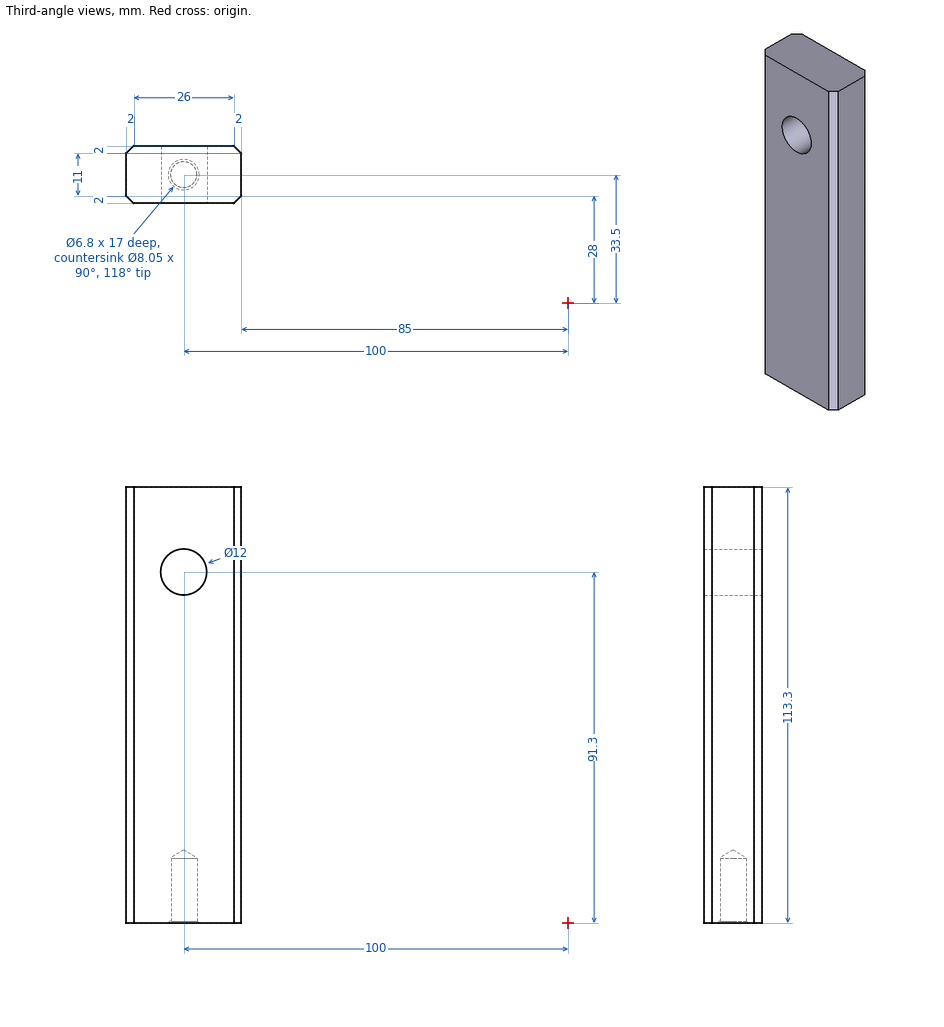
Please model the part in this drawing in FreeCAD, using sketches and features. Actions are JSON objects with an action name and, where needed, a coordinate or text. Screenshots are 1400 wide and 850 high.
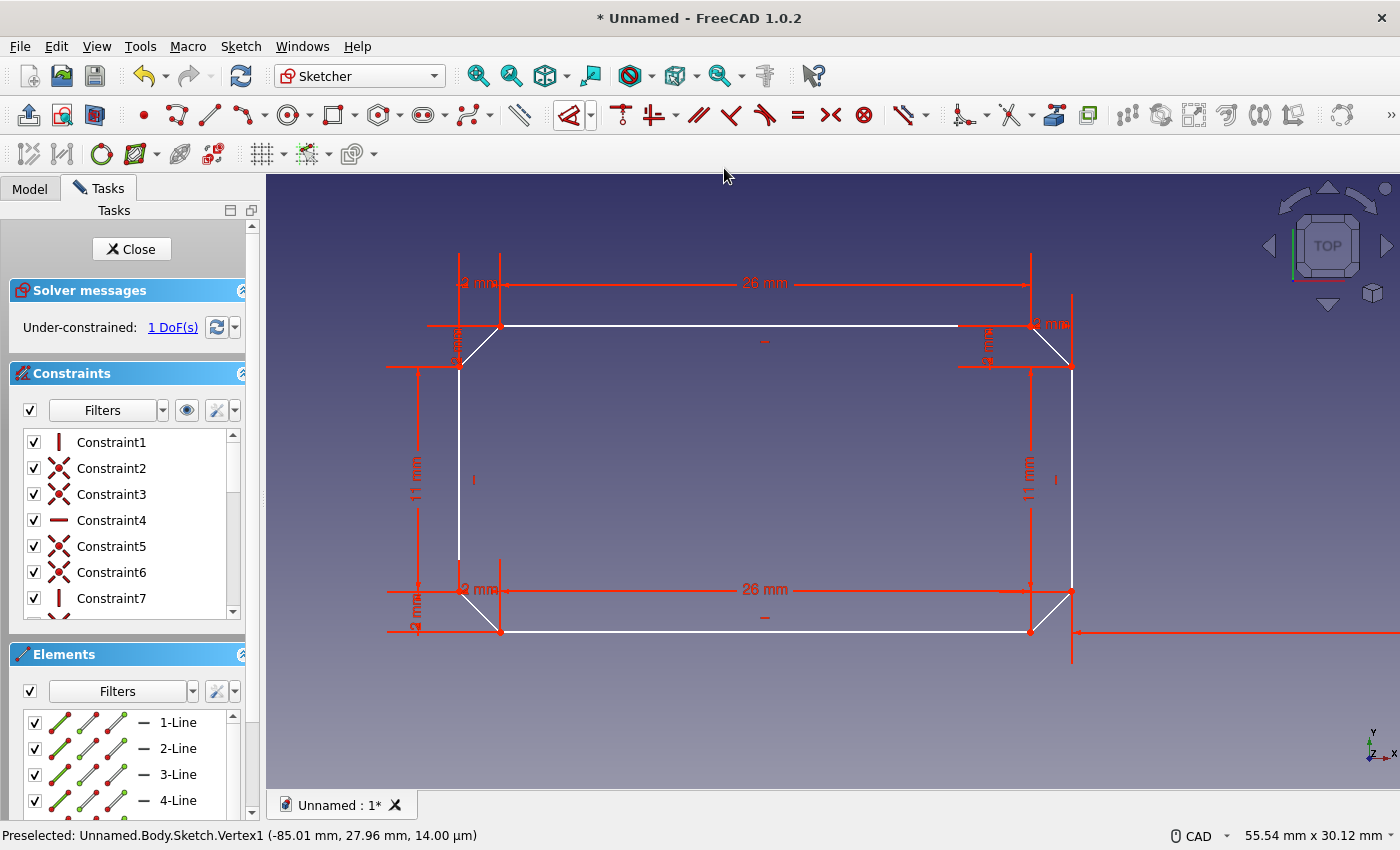
{"action": "left_click", "coordinate": [1072, 592]}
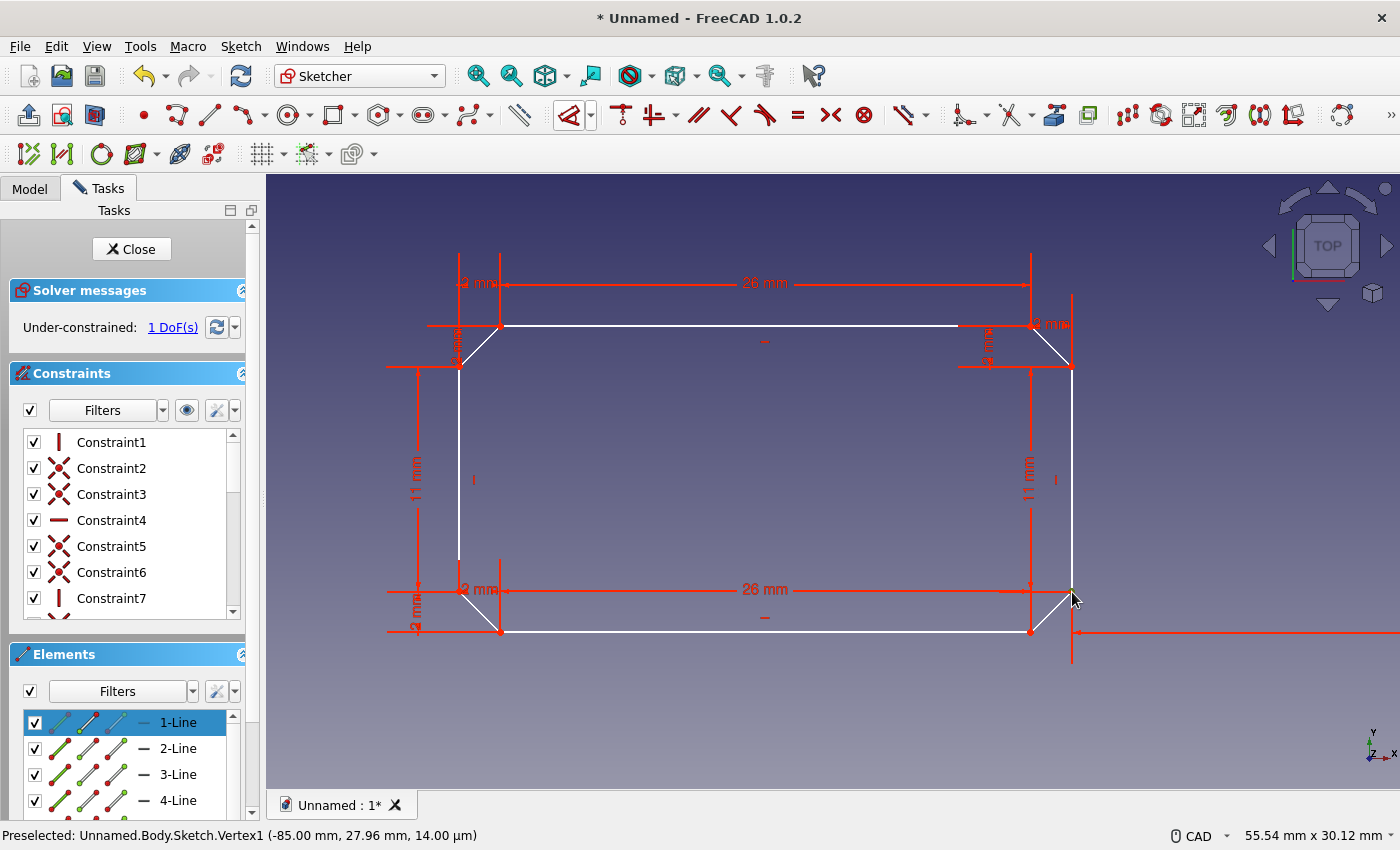
{"action": "left_click", "coordinate": [590, 116]}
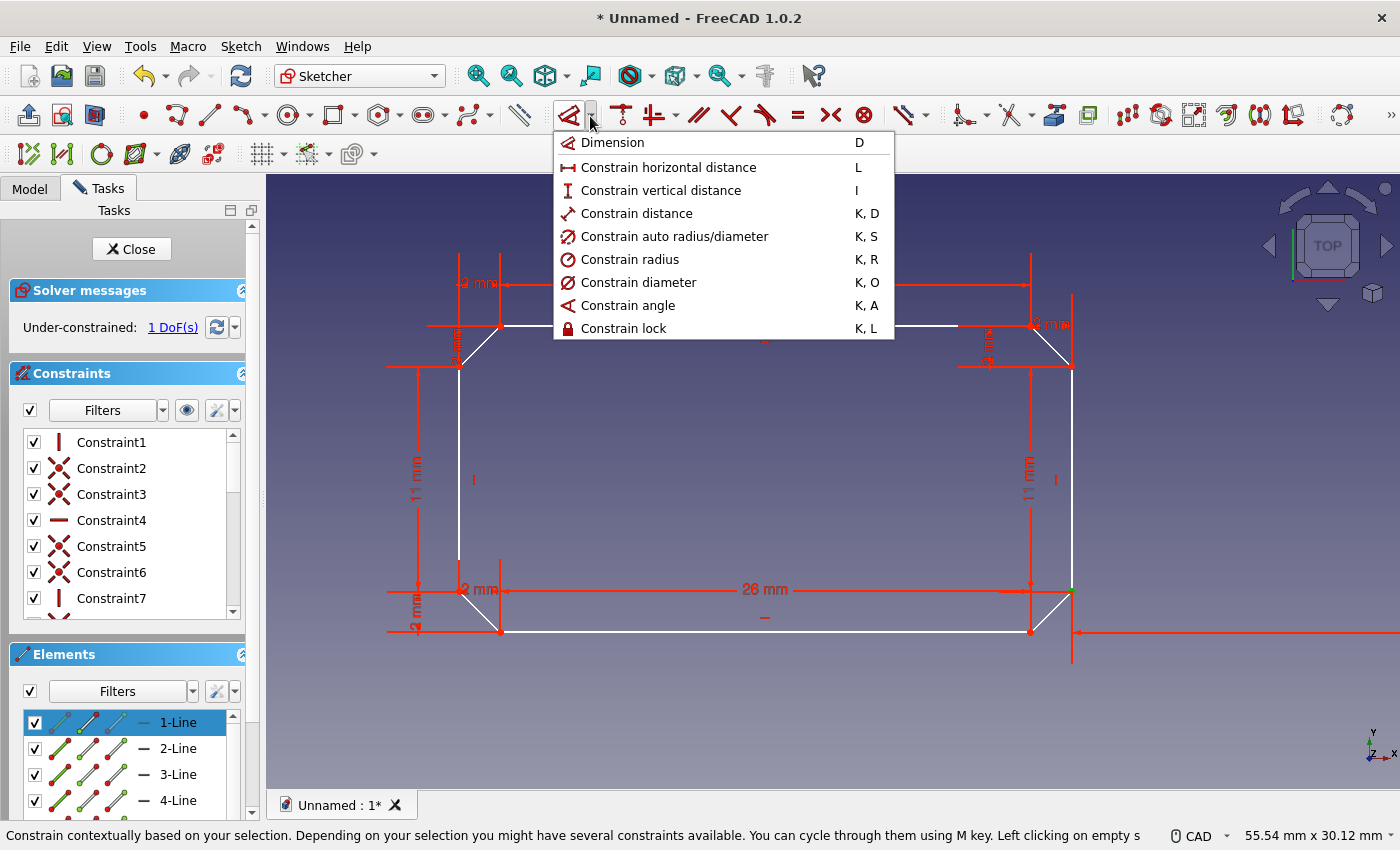
{"action": "left_click", "coordinate": [724, 190]}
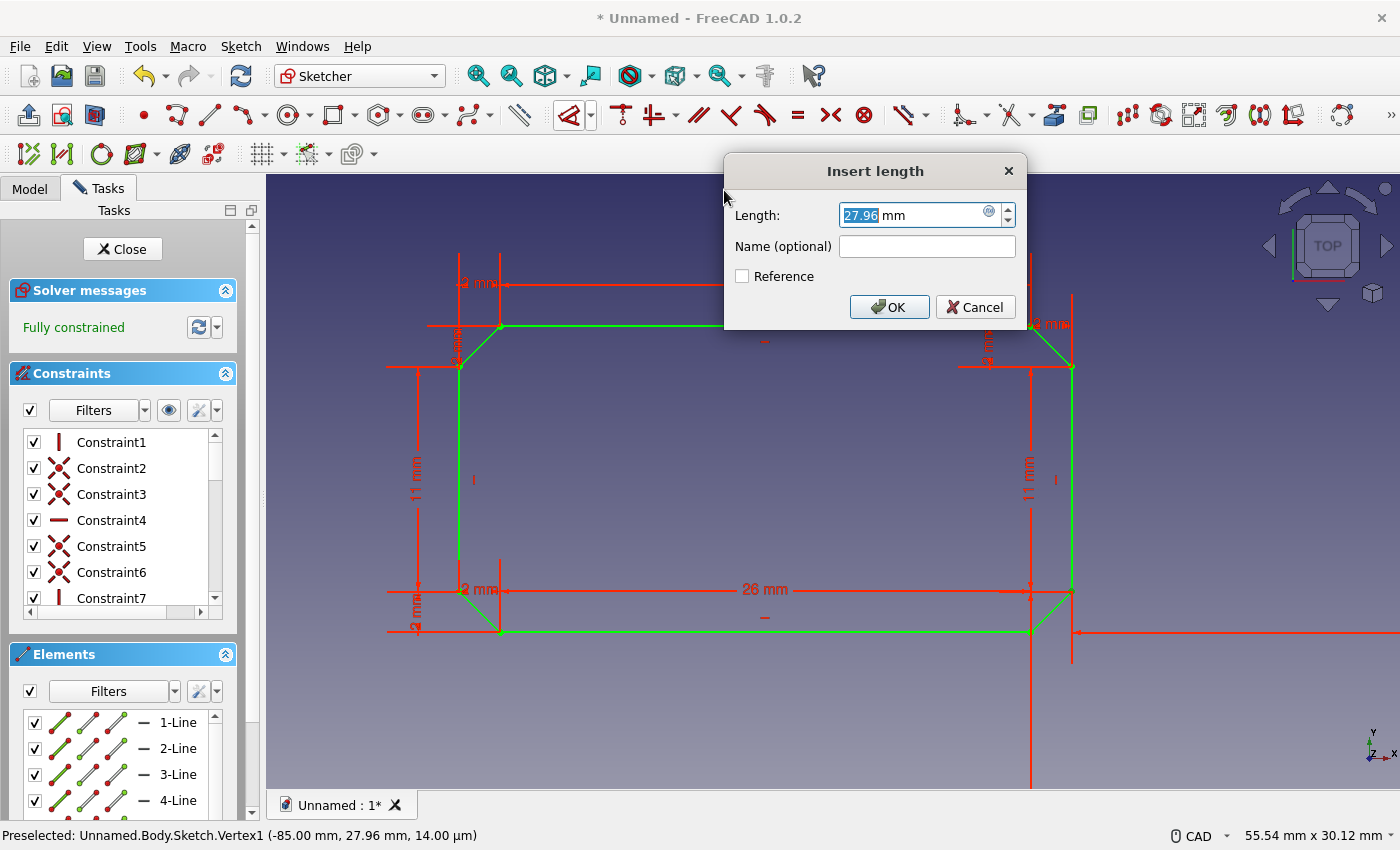
{"action": "type", "text": "28"}
{"action": "key", "text": "Return"}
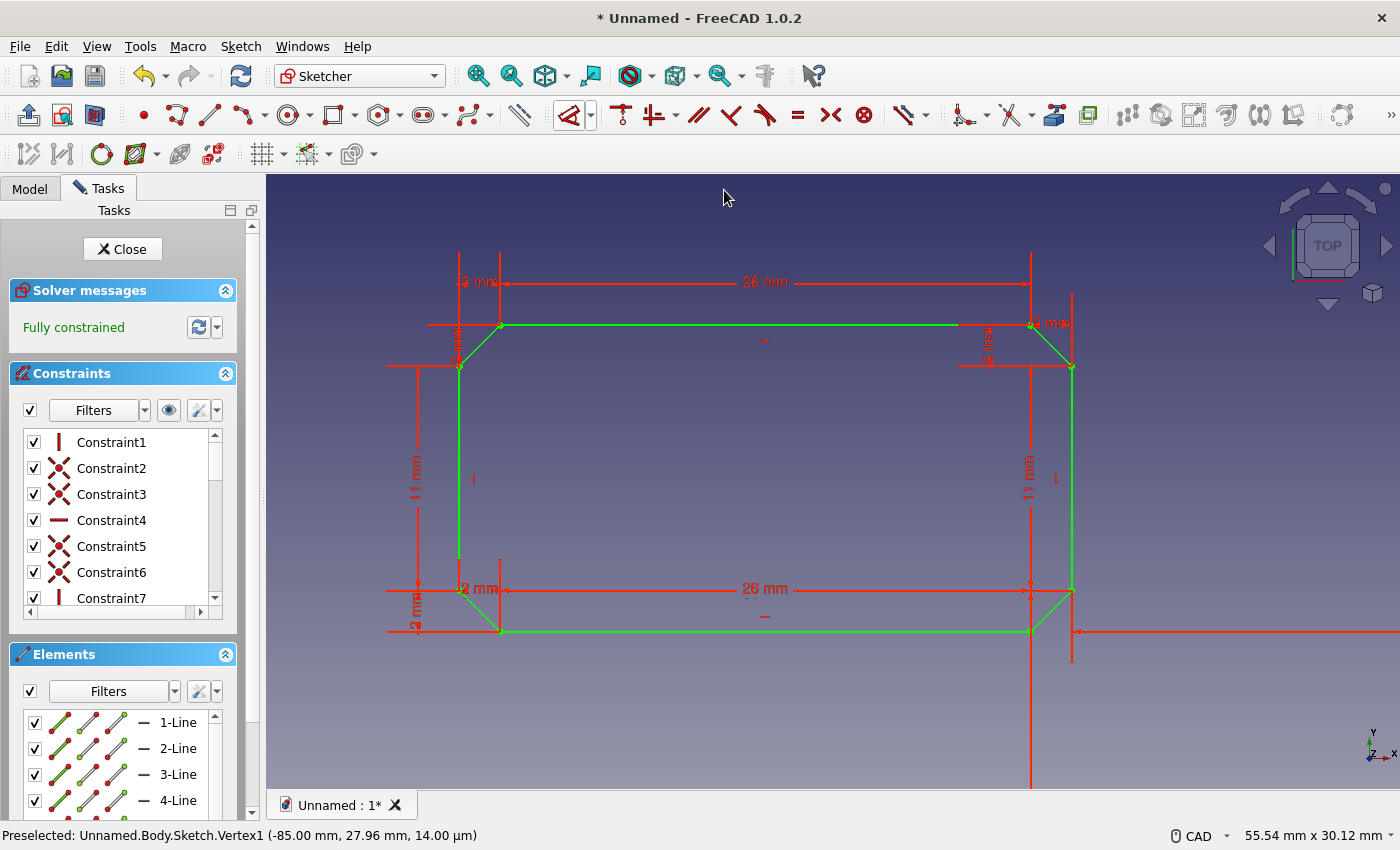
{"action": "left_click", "coordinate": [123, 249]}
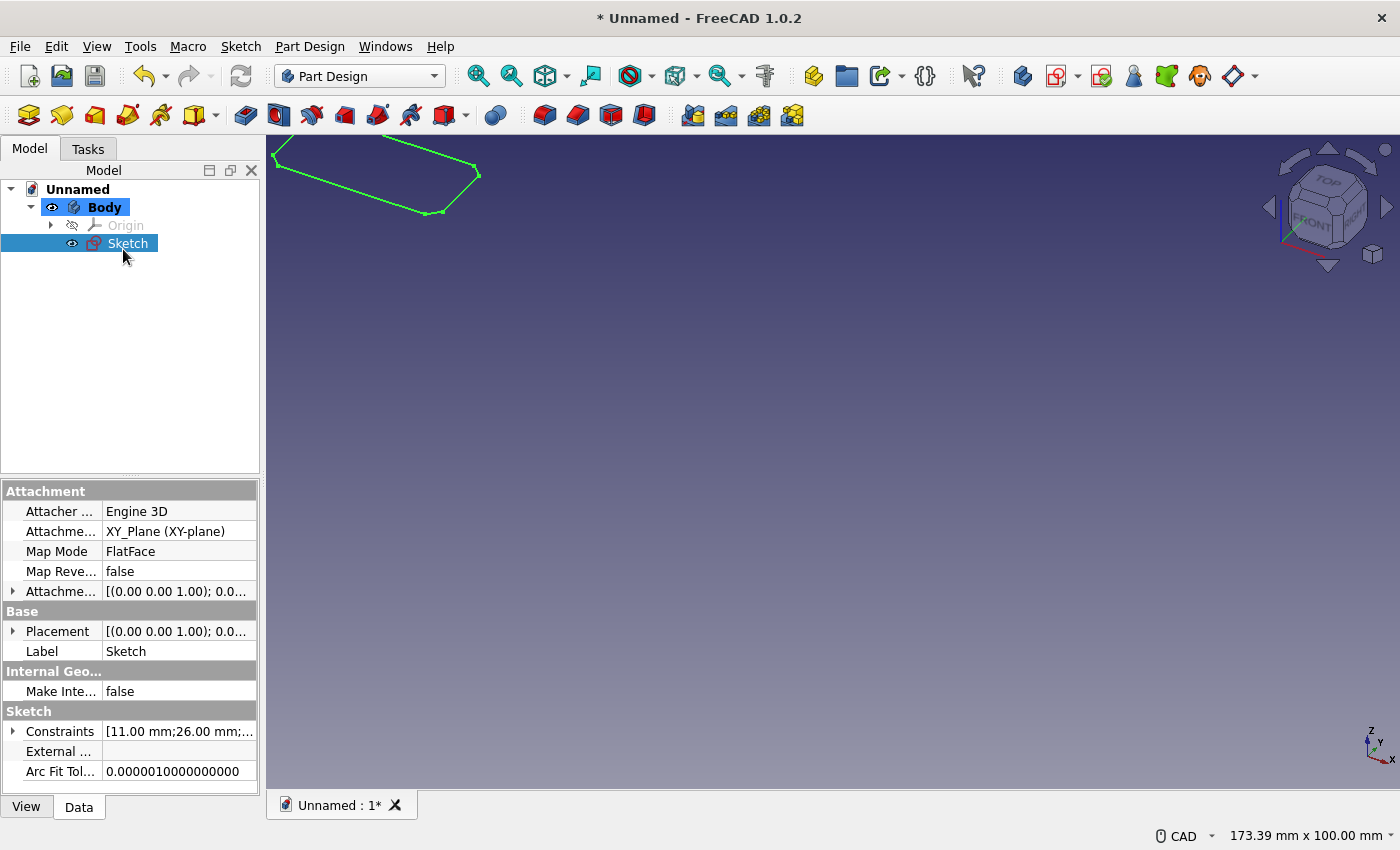
{"action": "left_click", "coordinate": [29, 116]}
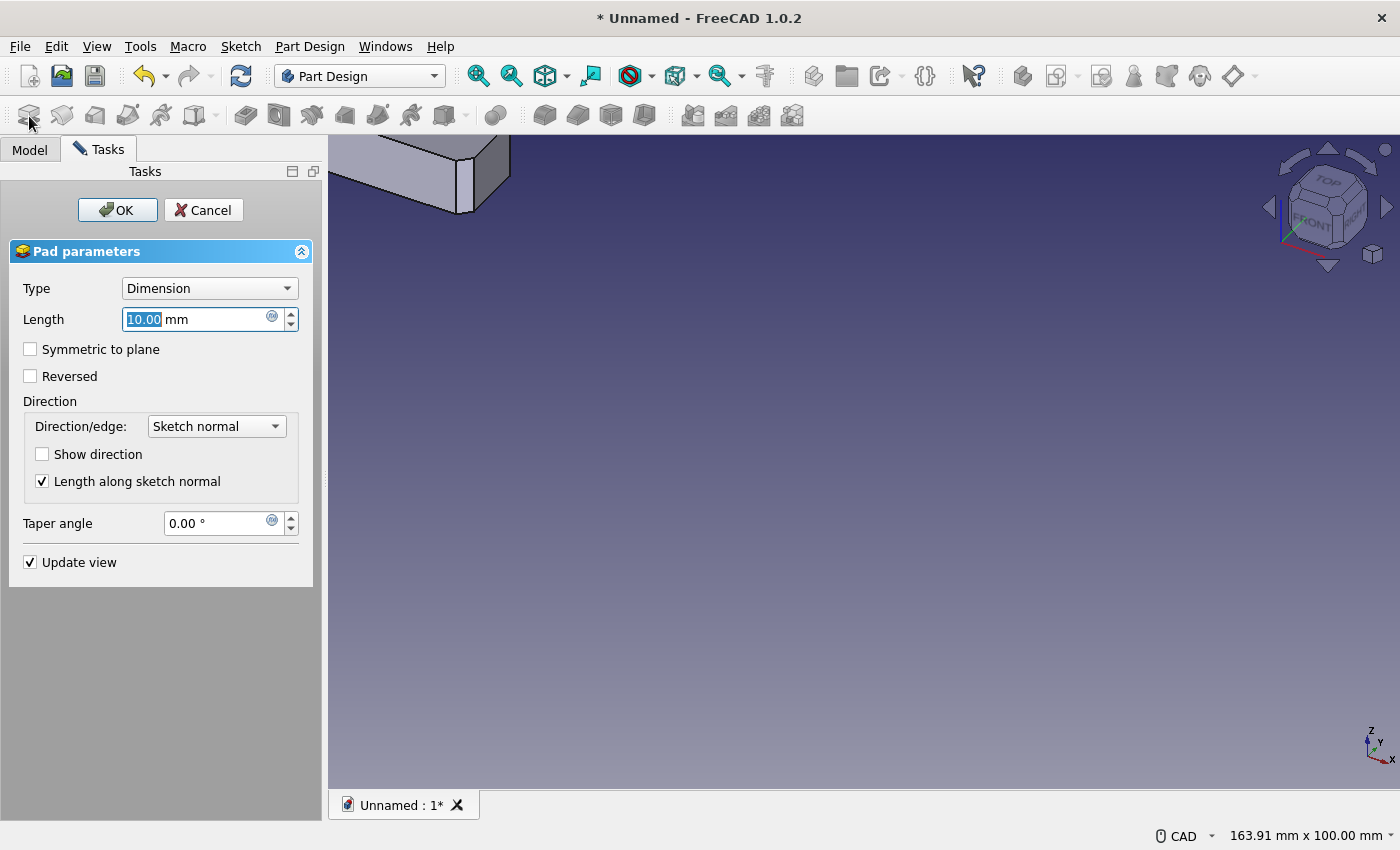
{"action": "type", "text": "113.3"}
{"action": "key", "text": "Tab"}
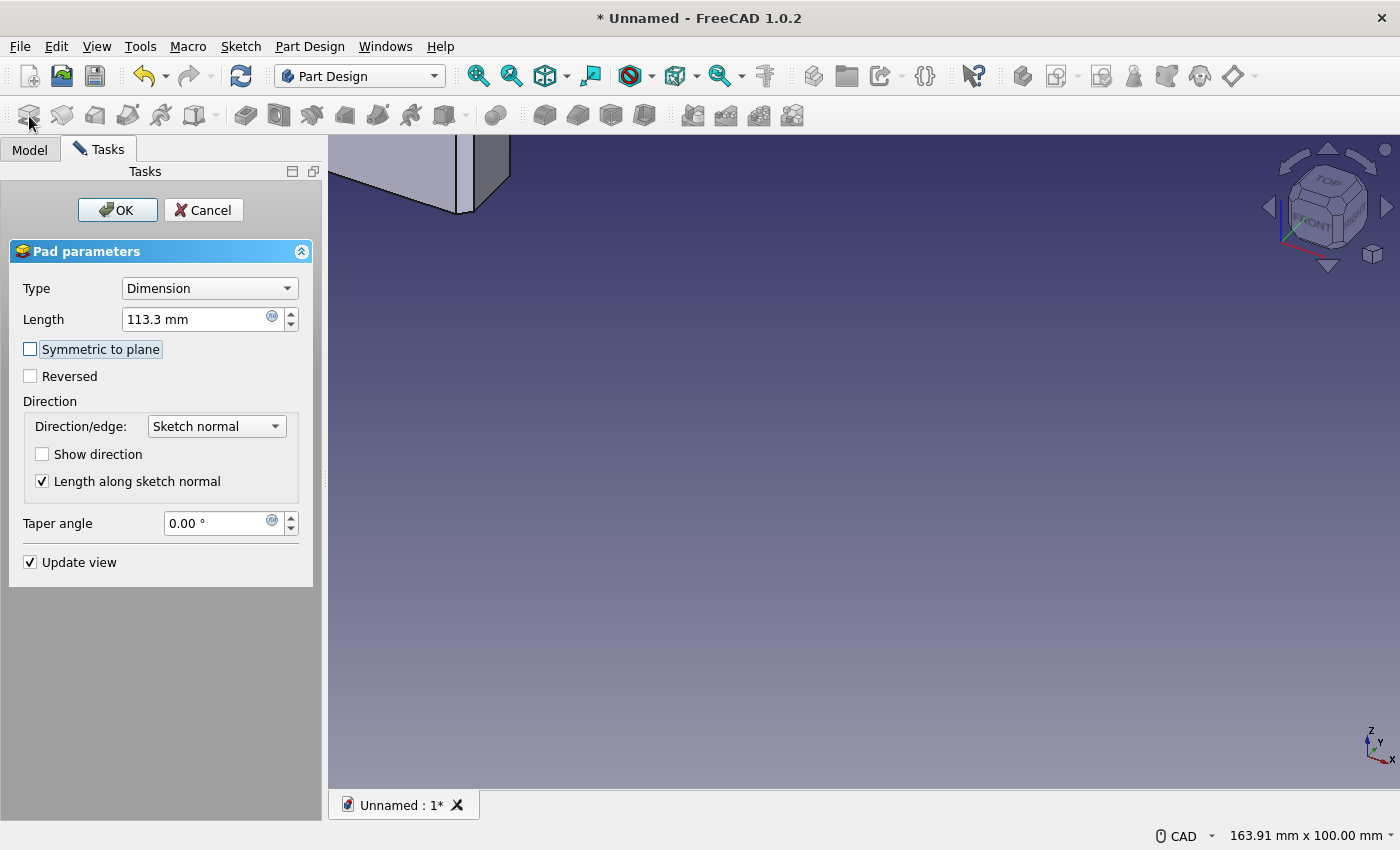
{"action": "left_click", "coordinate": [118, 210]}